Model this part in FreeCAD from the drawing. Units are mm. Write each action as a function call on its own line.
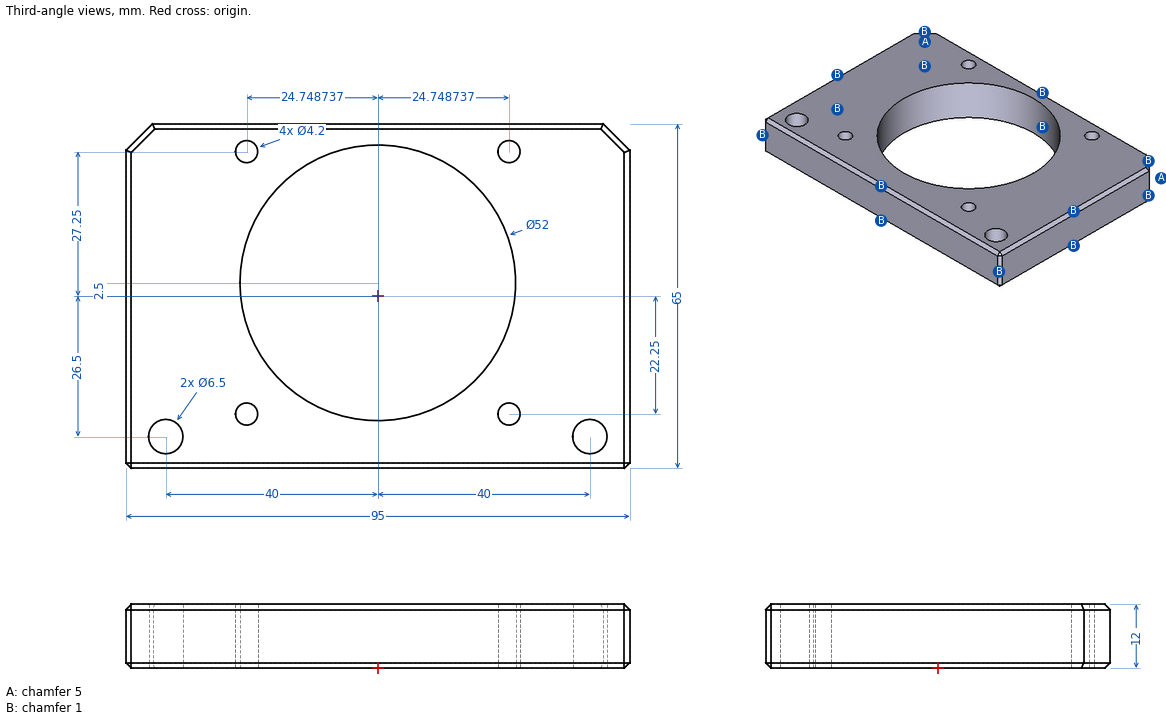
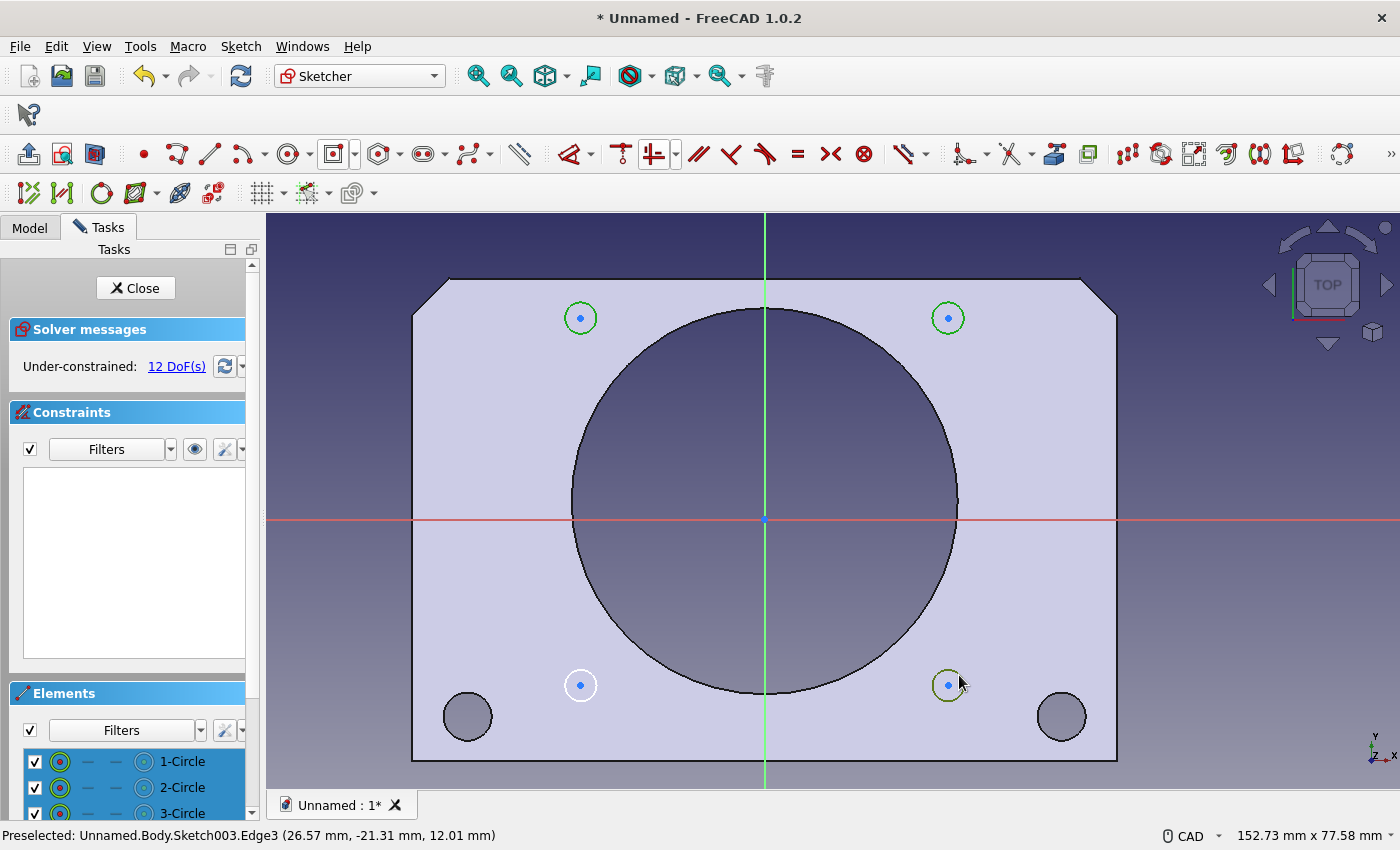
click(592, 675)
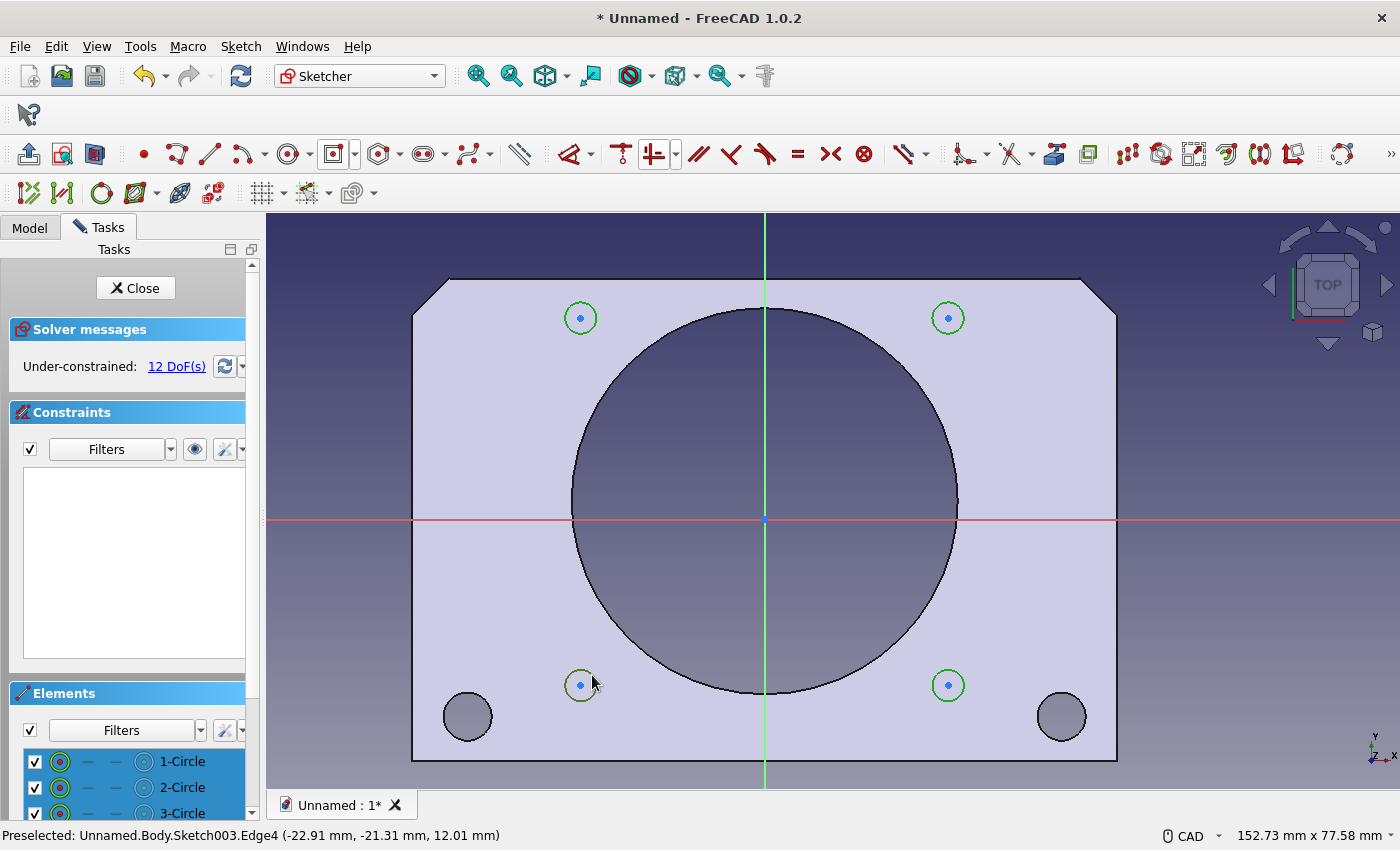
click(798, 154)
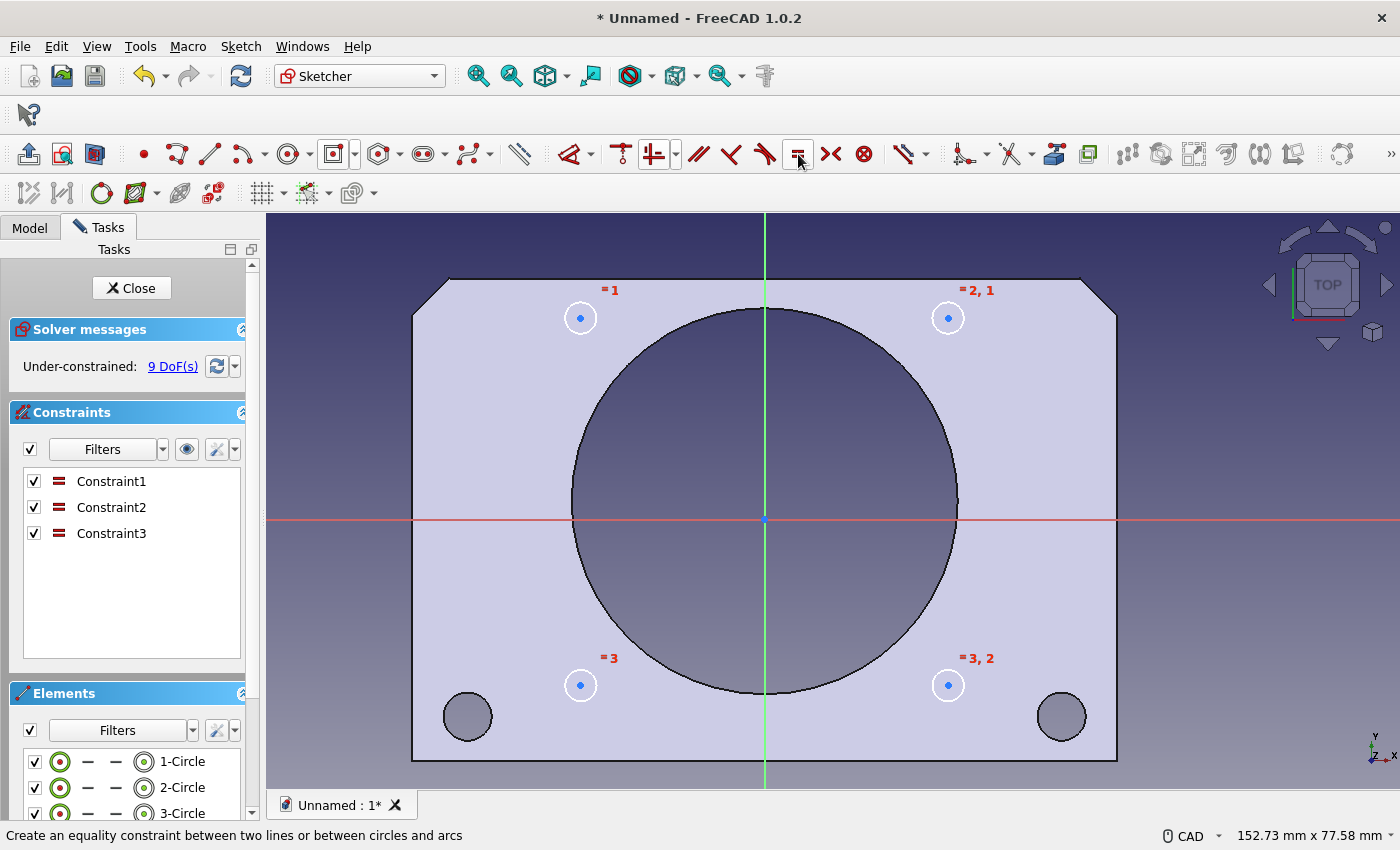
click(581, 318)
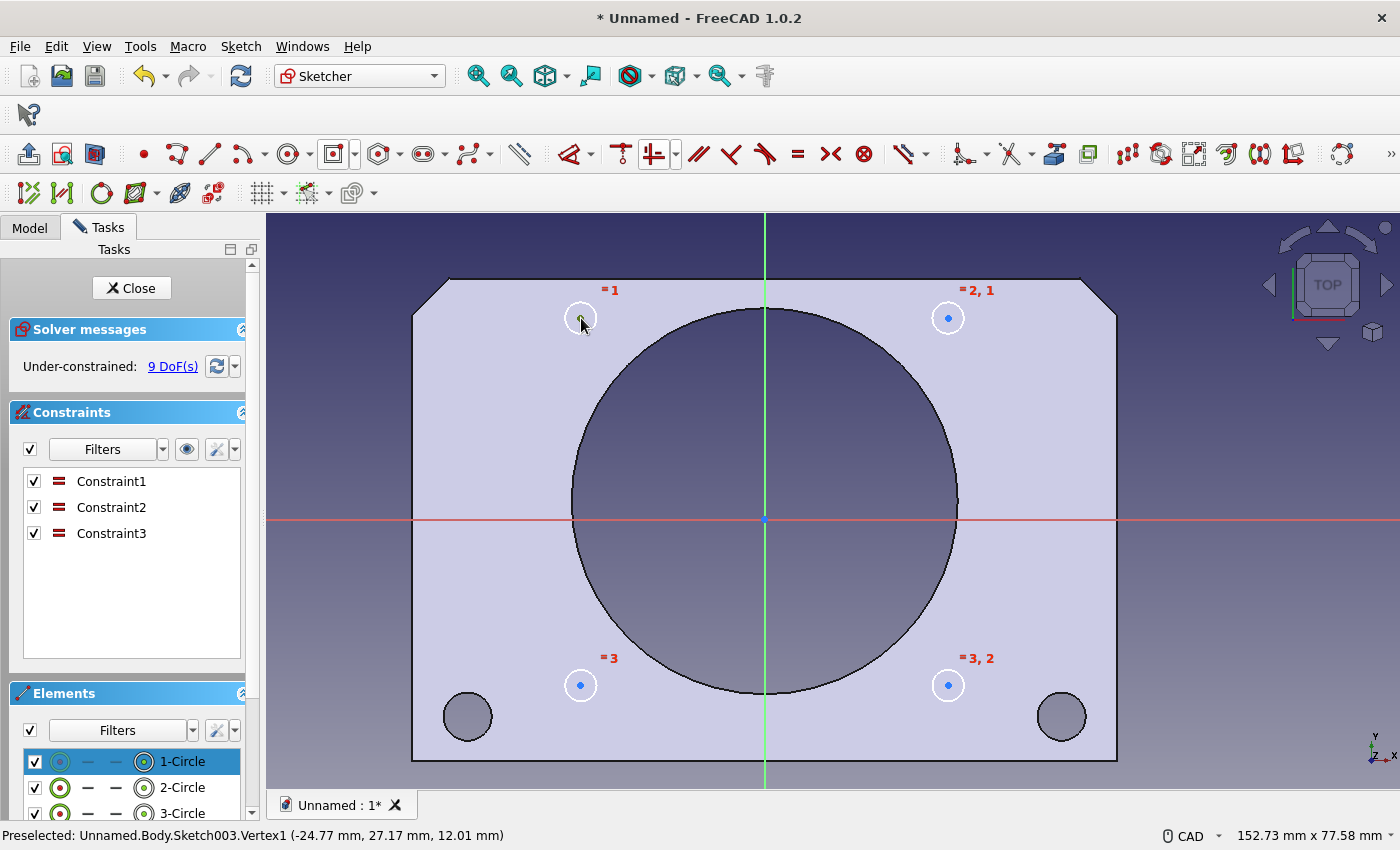
click(948, 318)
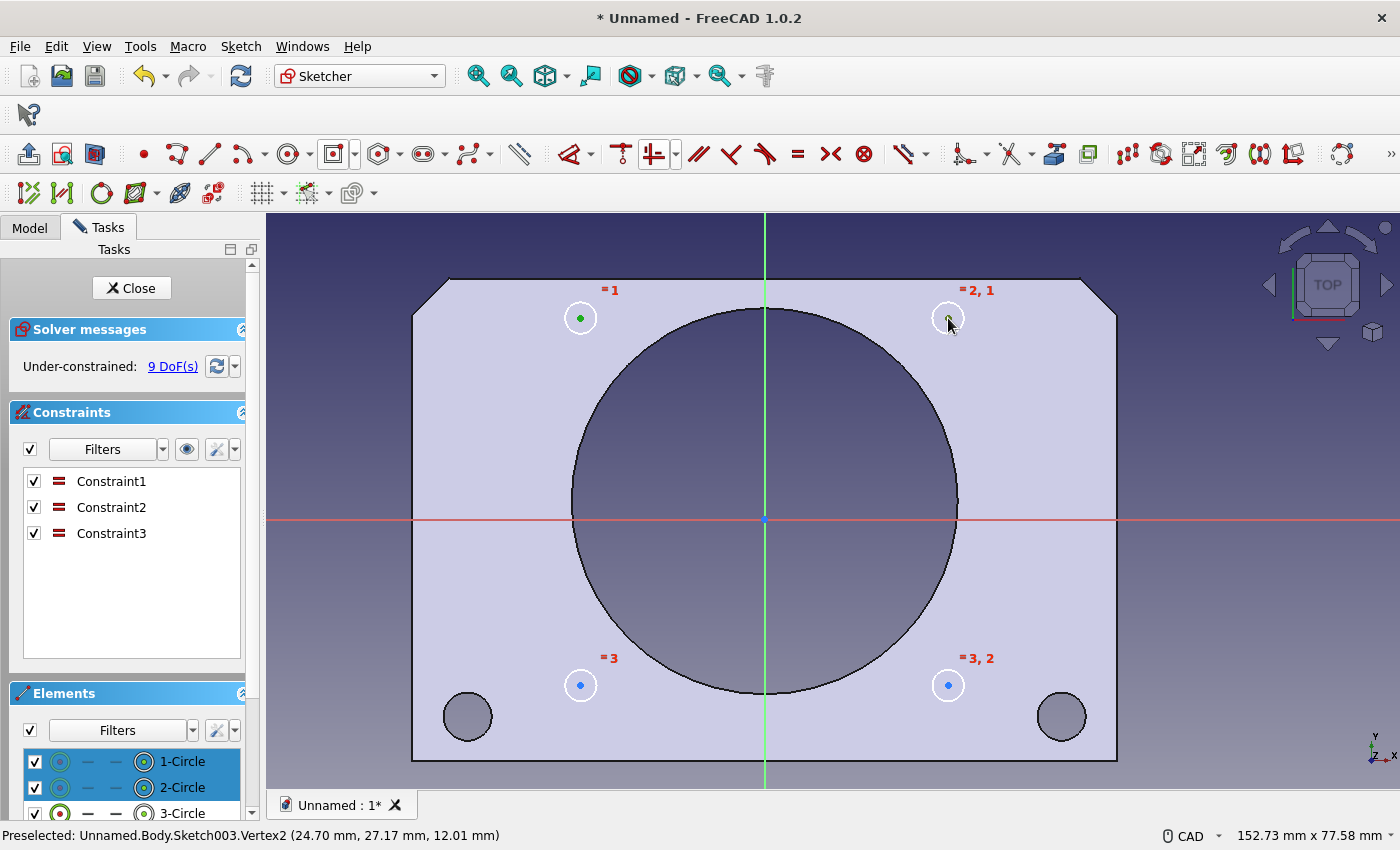
key(h)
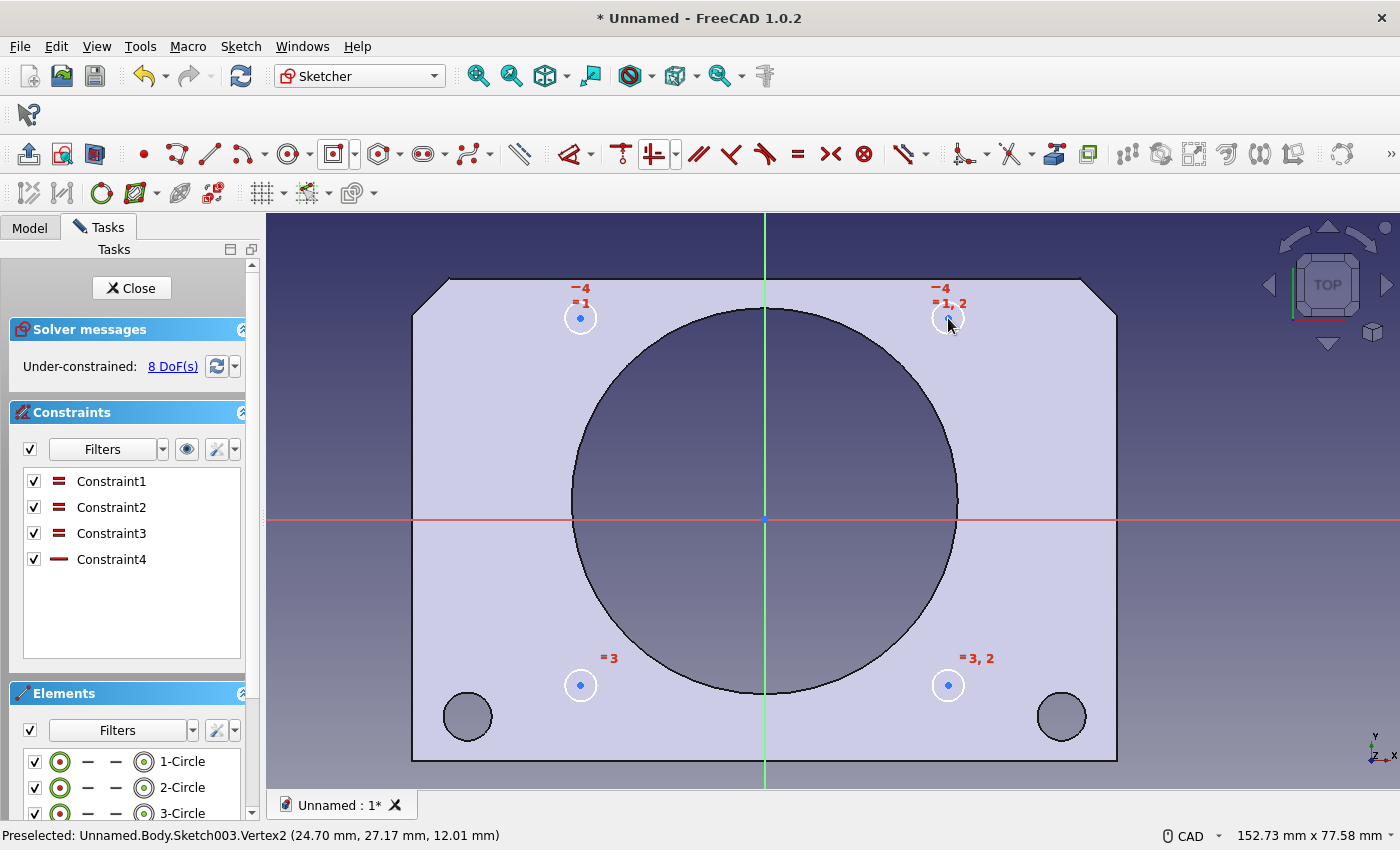
click(948, 318)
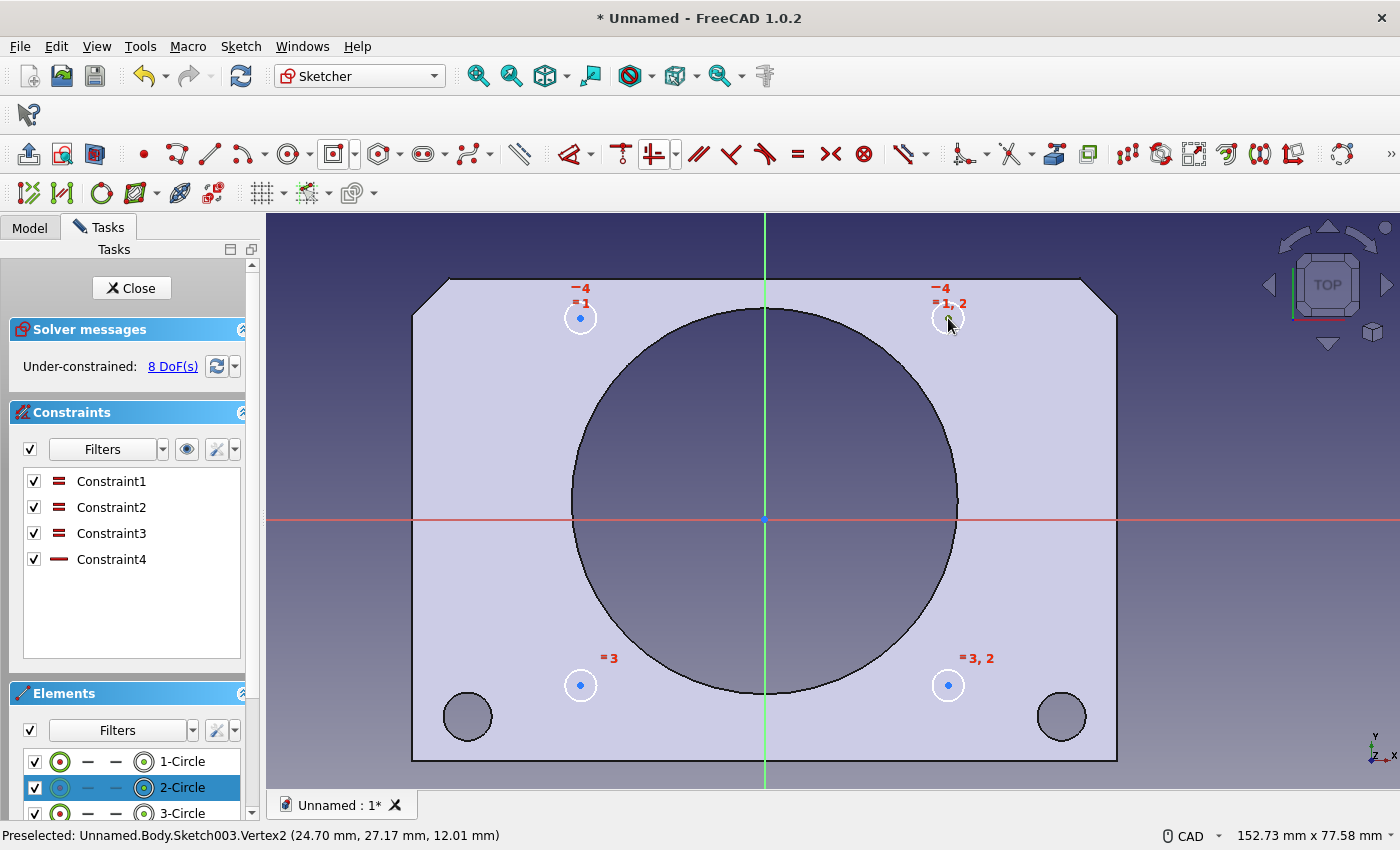
click(948, 686)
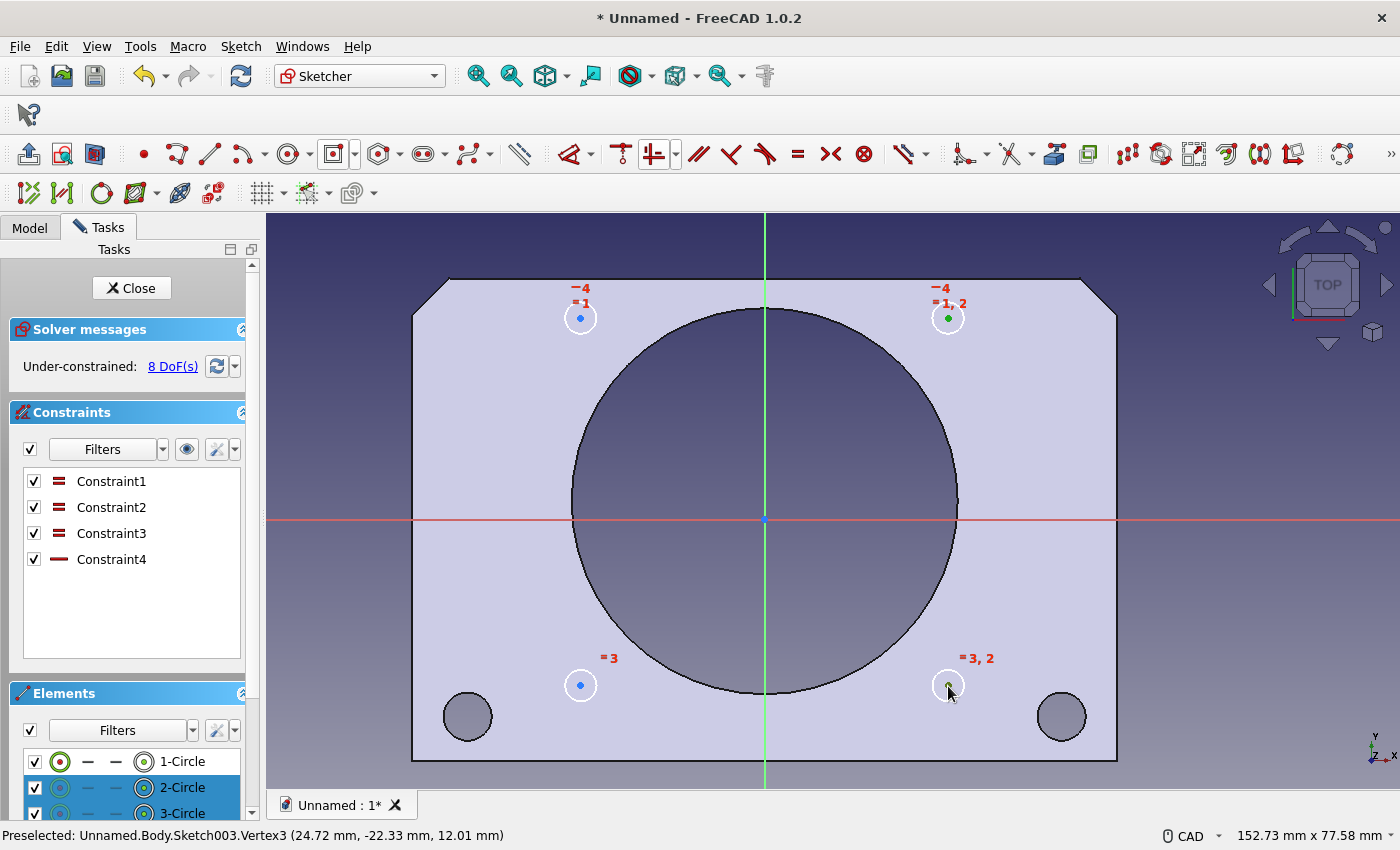
click(676, 154)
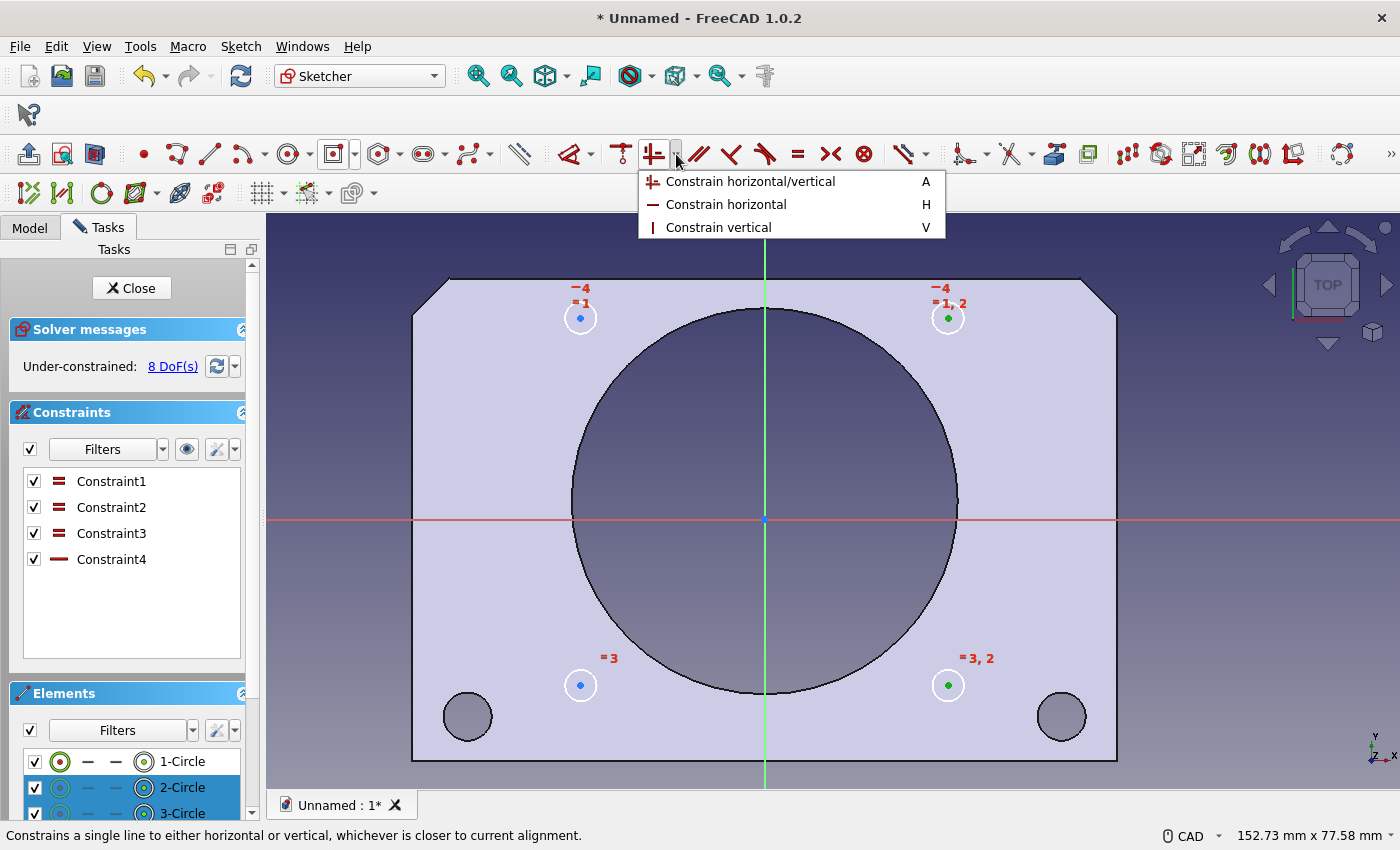
click(792, 228)